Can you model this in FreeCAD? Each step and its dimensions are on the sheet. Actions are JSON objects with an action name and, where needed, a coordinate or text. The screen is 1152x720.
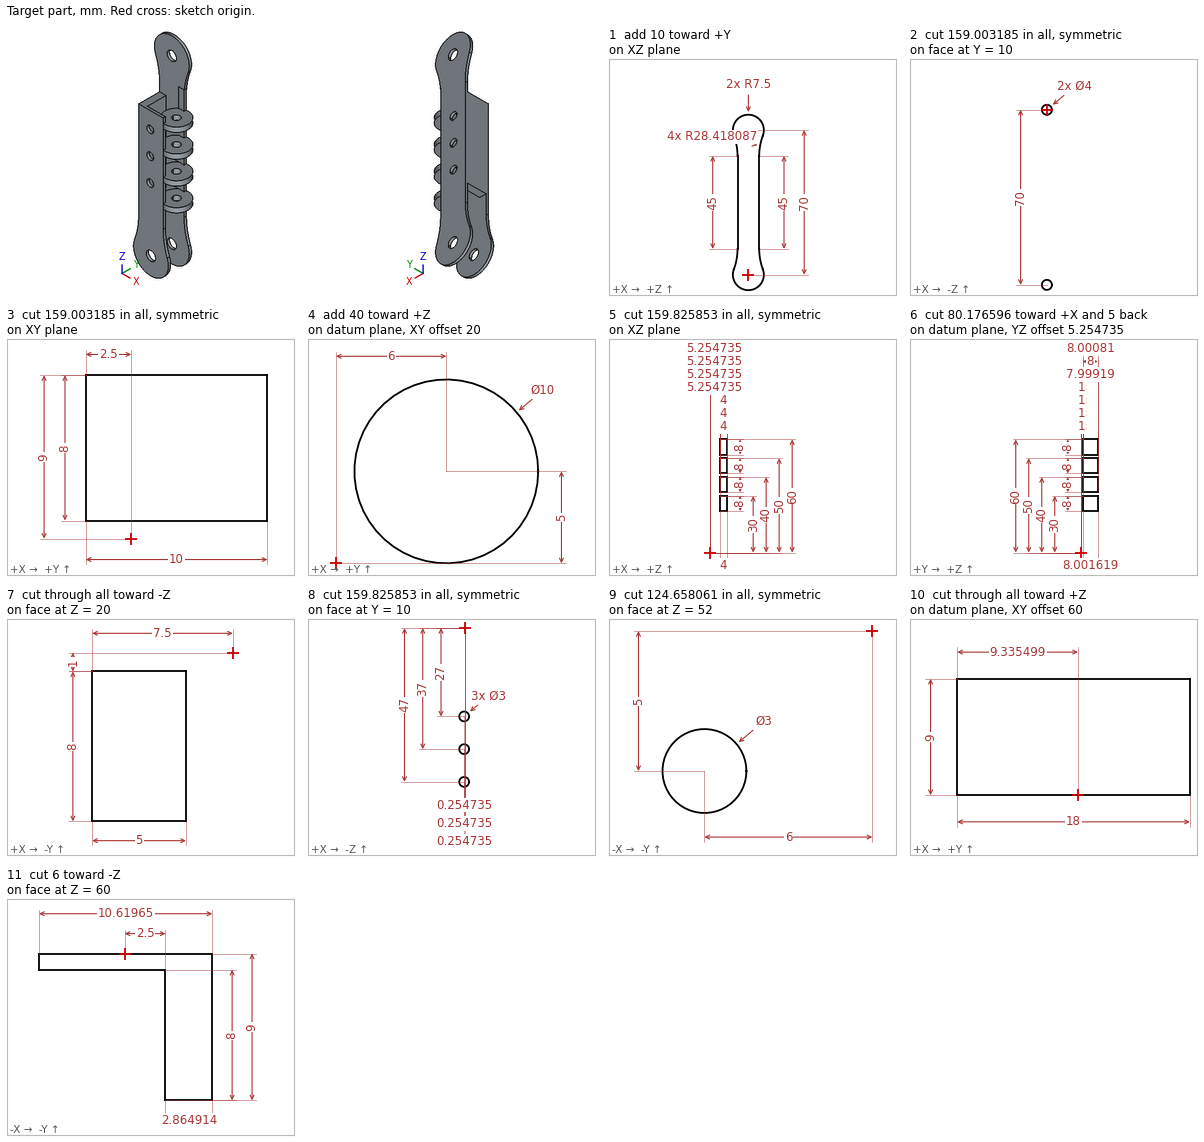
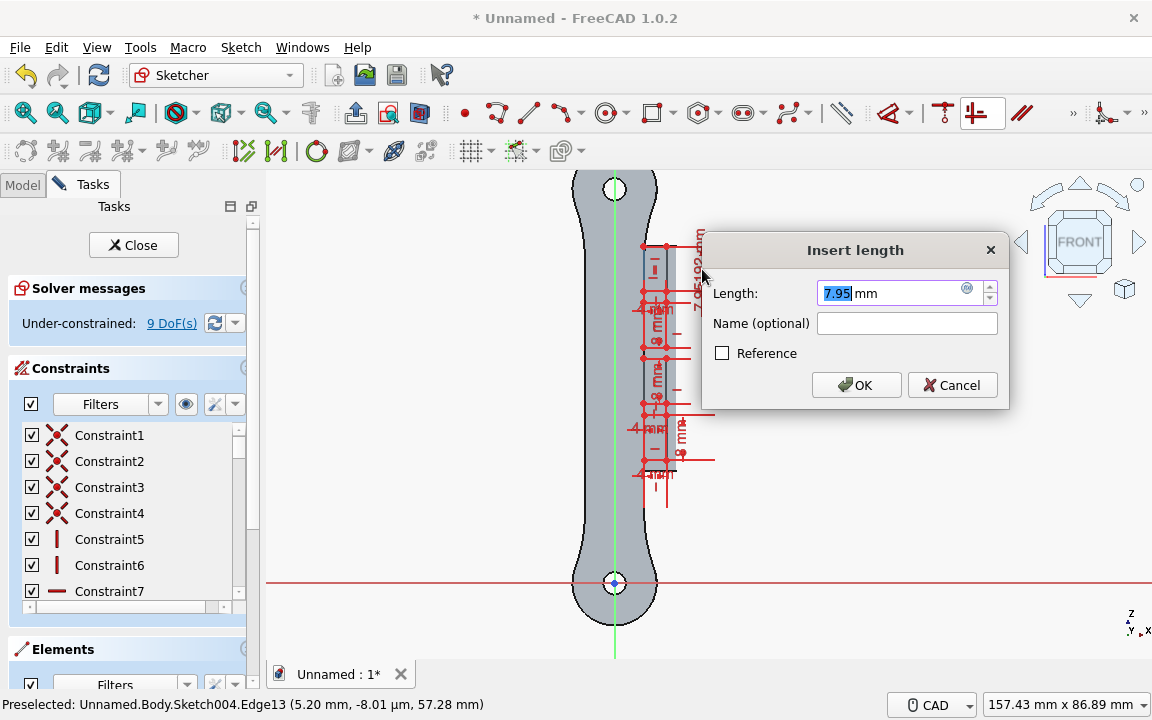
{"action": "type", "text": "8"}
{"action": "key", "text": "Return"}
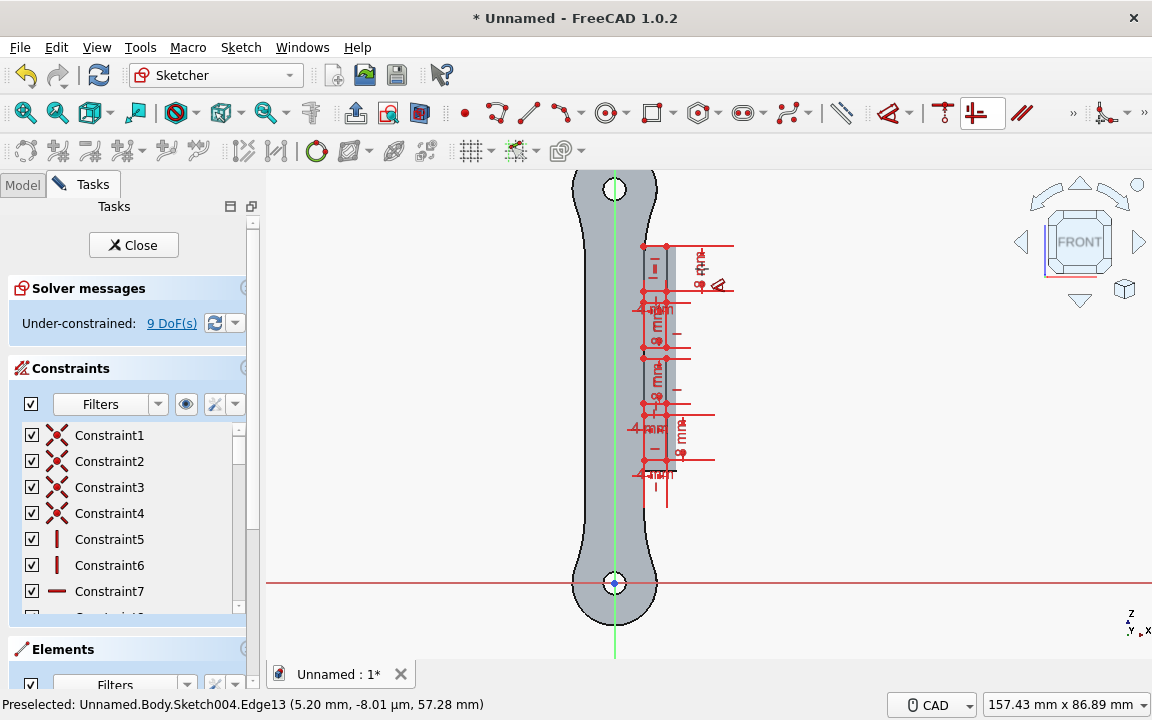
{"action": "scroll", "coordinate": [653, 291], "scroll_direction": "up", "scroll_amount": 3}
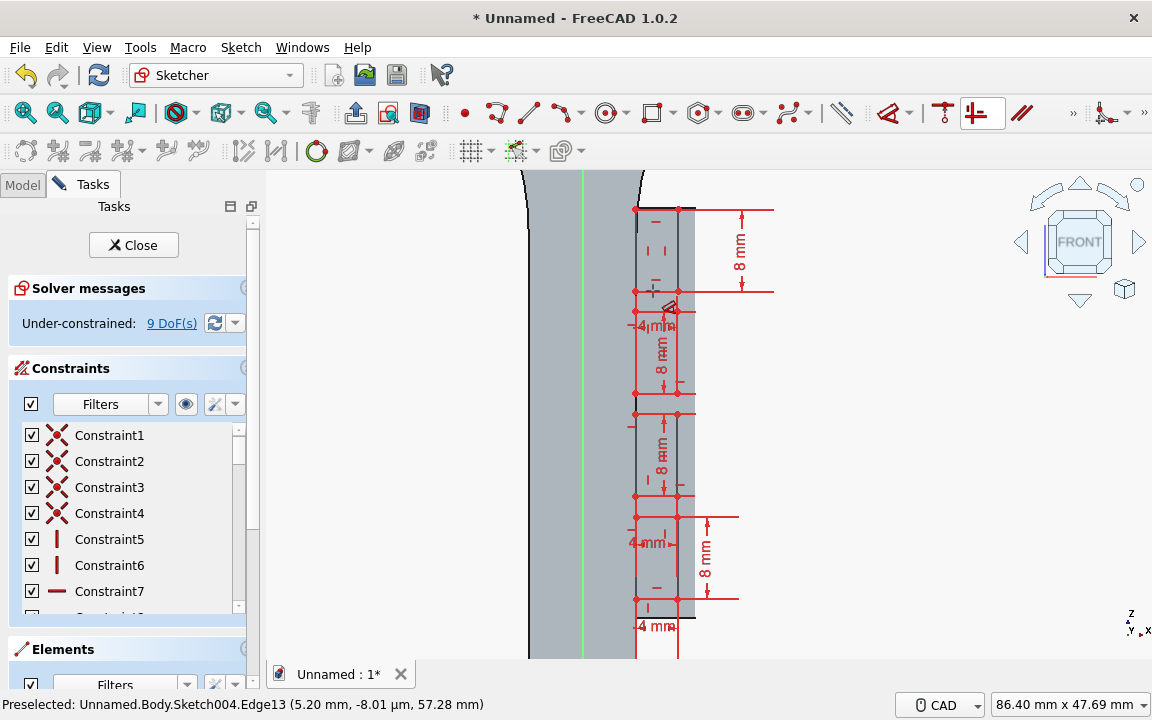
{"action": "left_click", "coordinate": [653, 292]}
{"action": "left_click", "coordinate": [657, 258]}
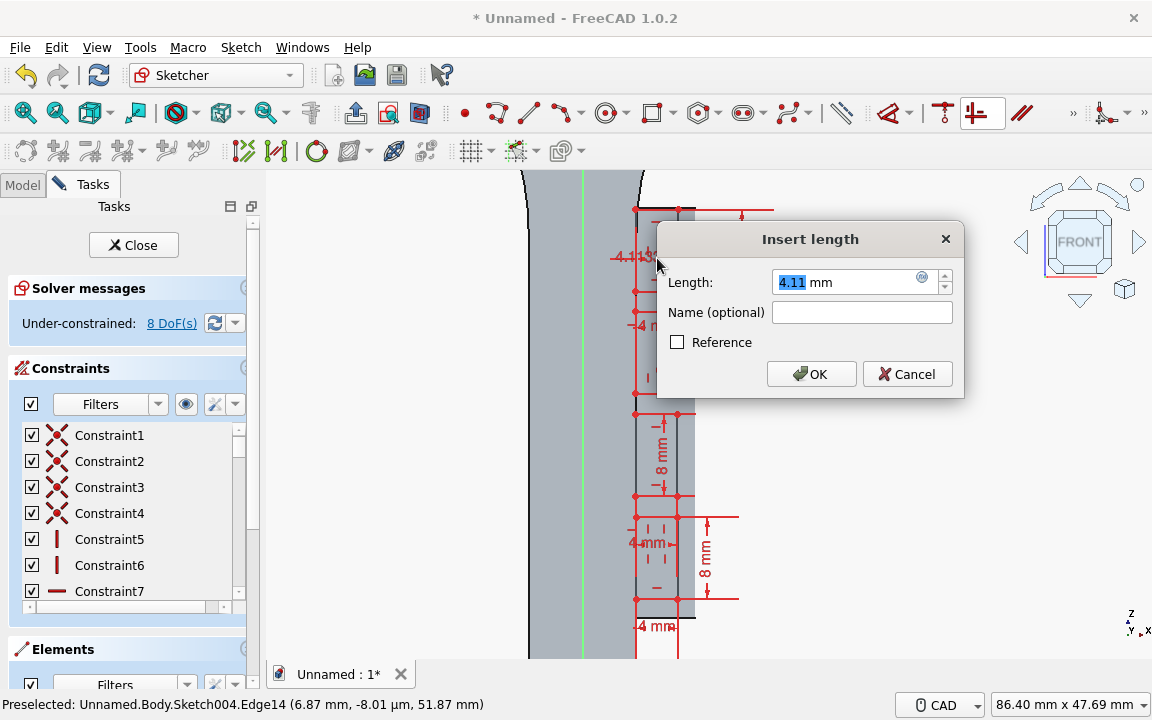
{"action": "type", "text": "4"}
{"action": "key", "text": "Return"}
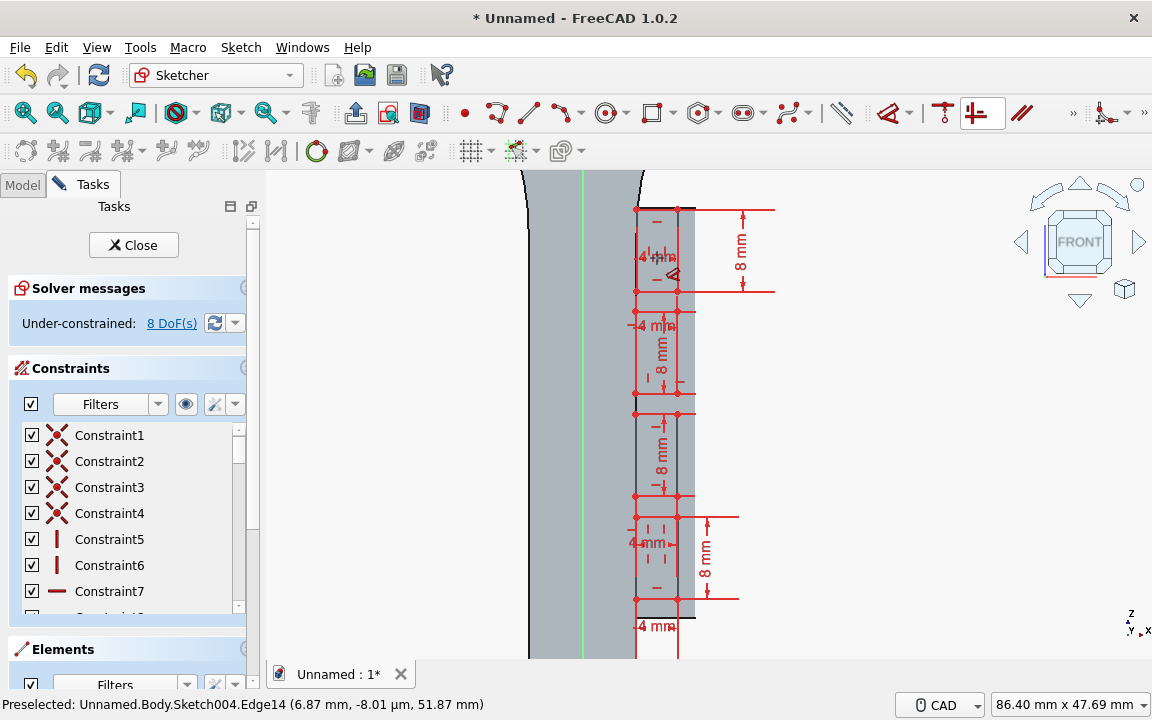
{"action": "left_click", "coordinate": [636, 517]}
{"action": "left_click", "coordinate": [549, 574]}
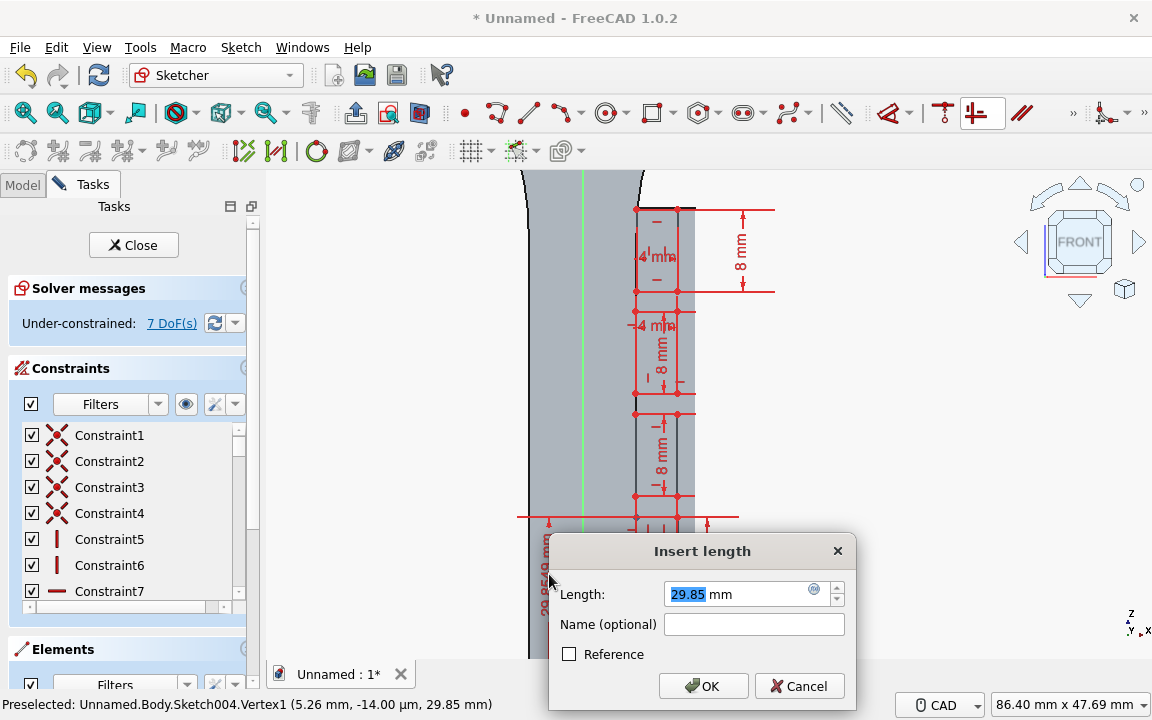
{"action": "type", "text": "30"}
{"action": "key", "text": "Return"}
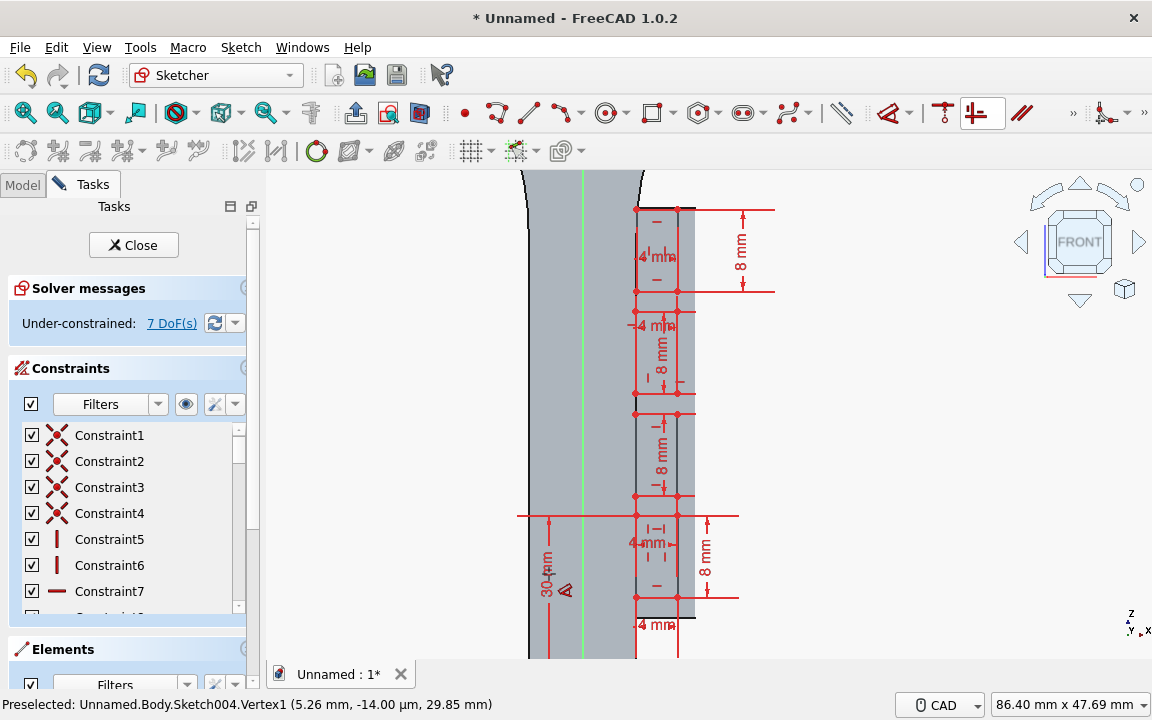
{"action": "left_click", "coordinate": [636, 414]}
{"action": "left_click", "coordinate": [549, 523]}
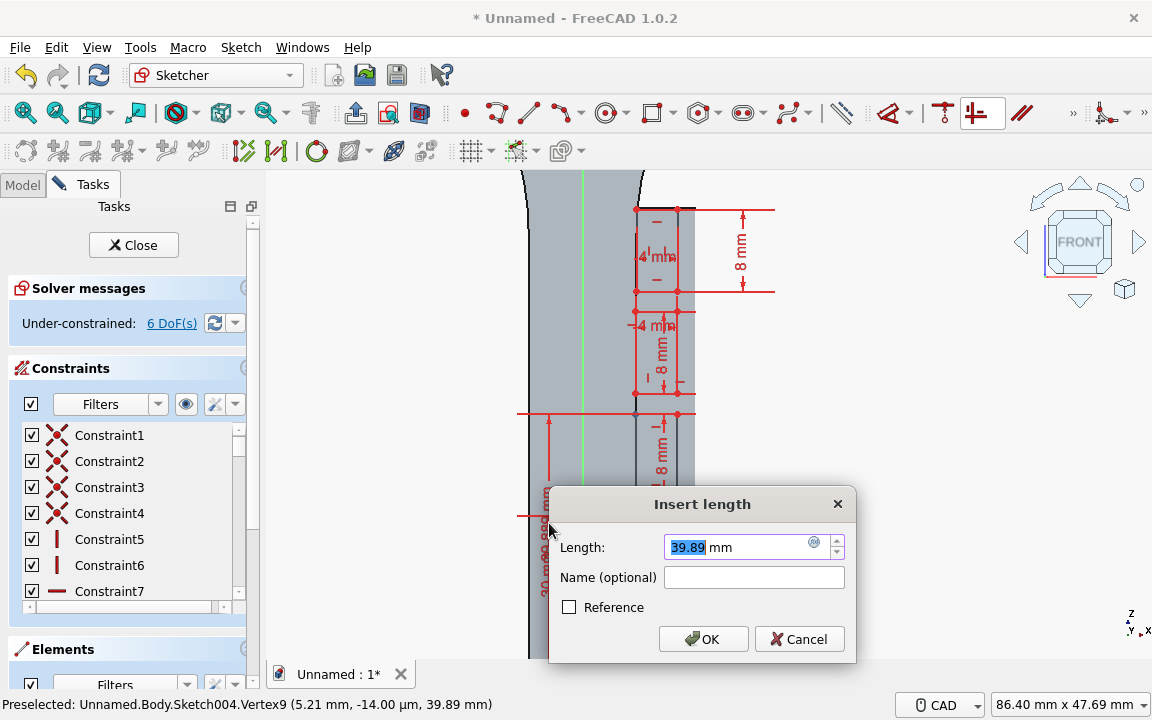
{"action": "type", "text": "40"}
{"action": "key", "text": "Return"}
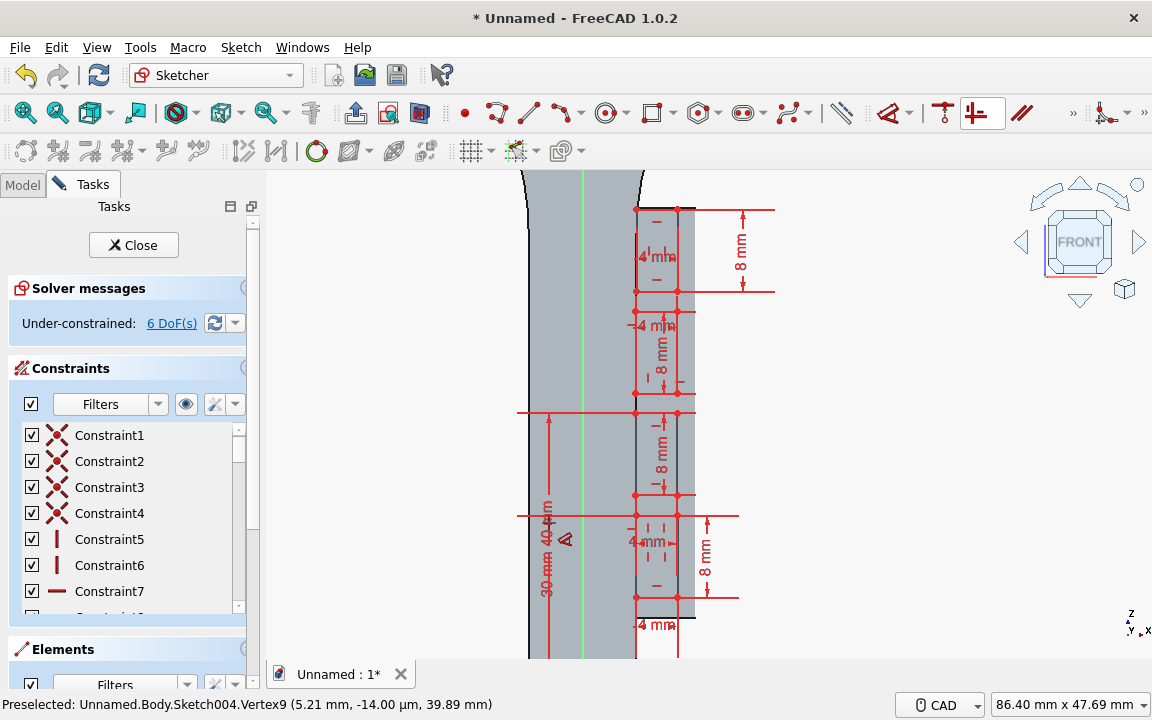
{"action": "left_click", "coordinate": [636, 312]}
{"action": "left_click", "coordinate": [549, 471]}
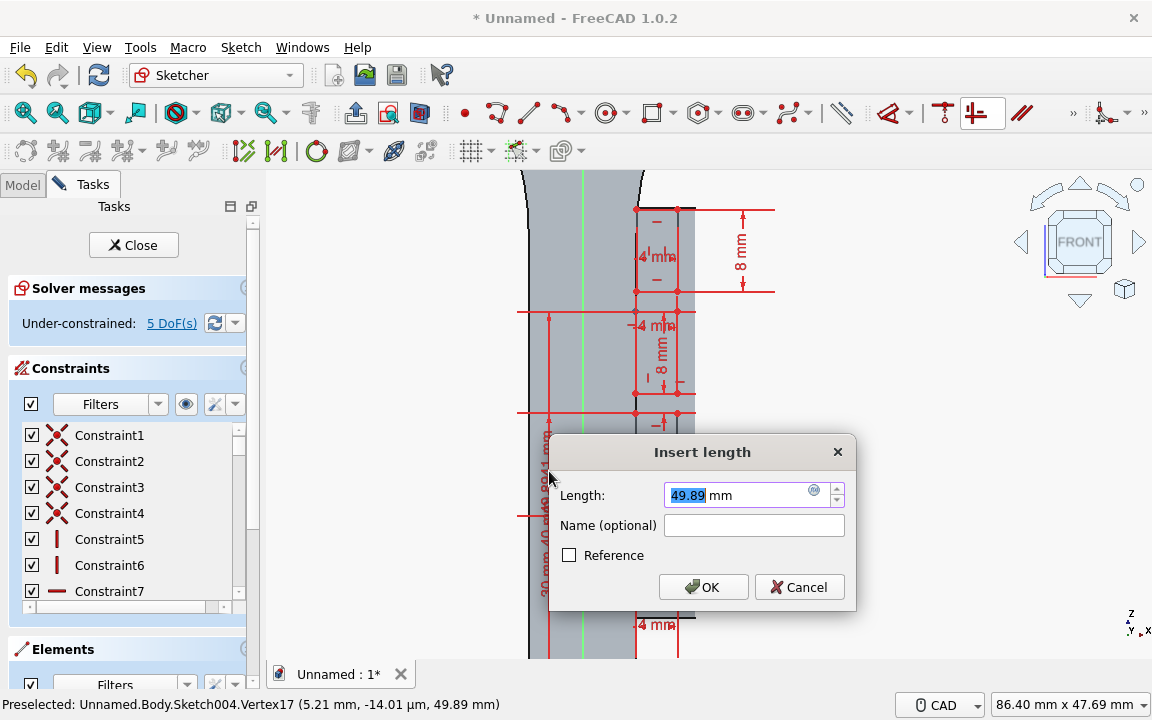
{"action": "type", "text": "50"}
{"action": "key", "text": "Return"}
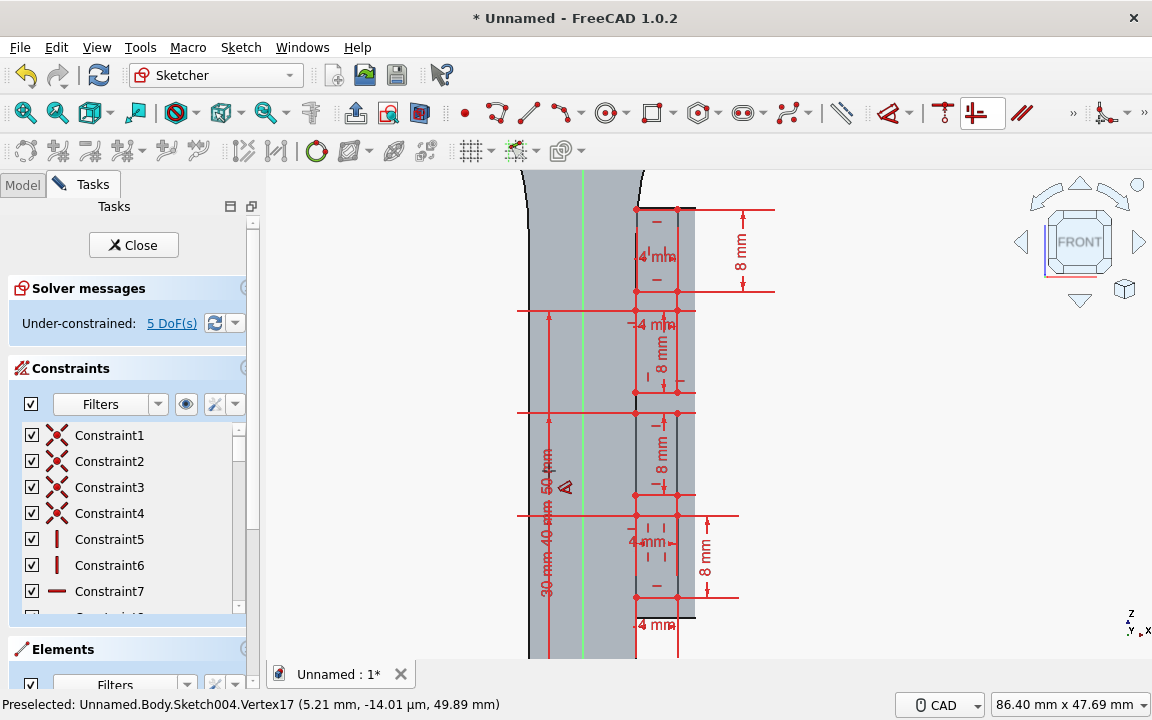
{"action": "left_click", "coordinate": [637, 210]}
{"action": "left_click", "coordinate": [549, 420]}